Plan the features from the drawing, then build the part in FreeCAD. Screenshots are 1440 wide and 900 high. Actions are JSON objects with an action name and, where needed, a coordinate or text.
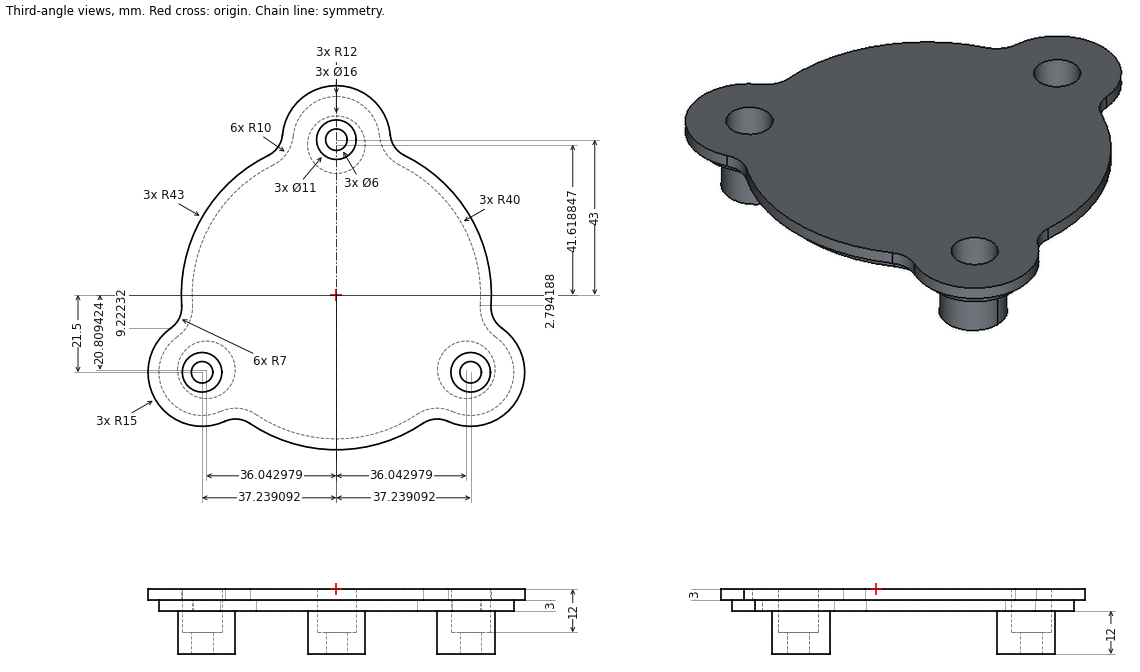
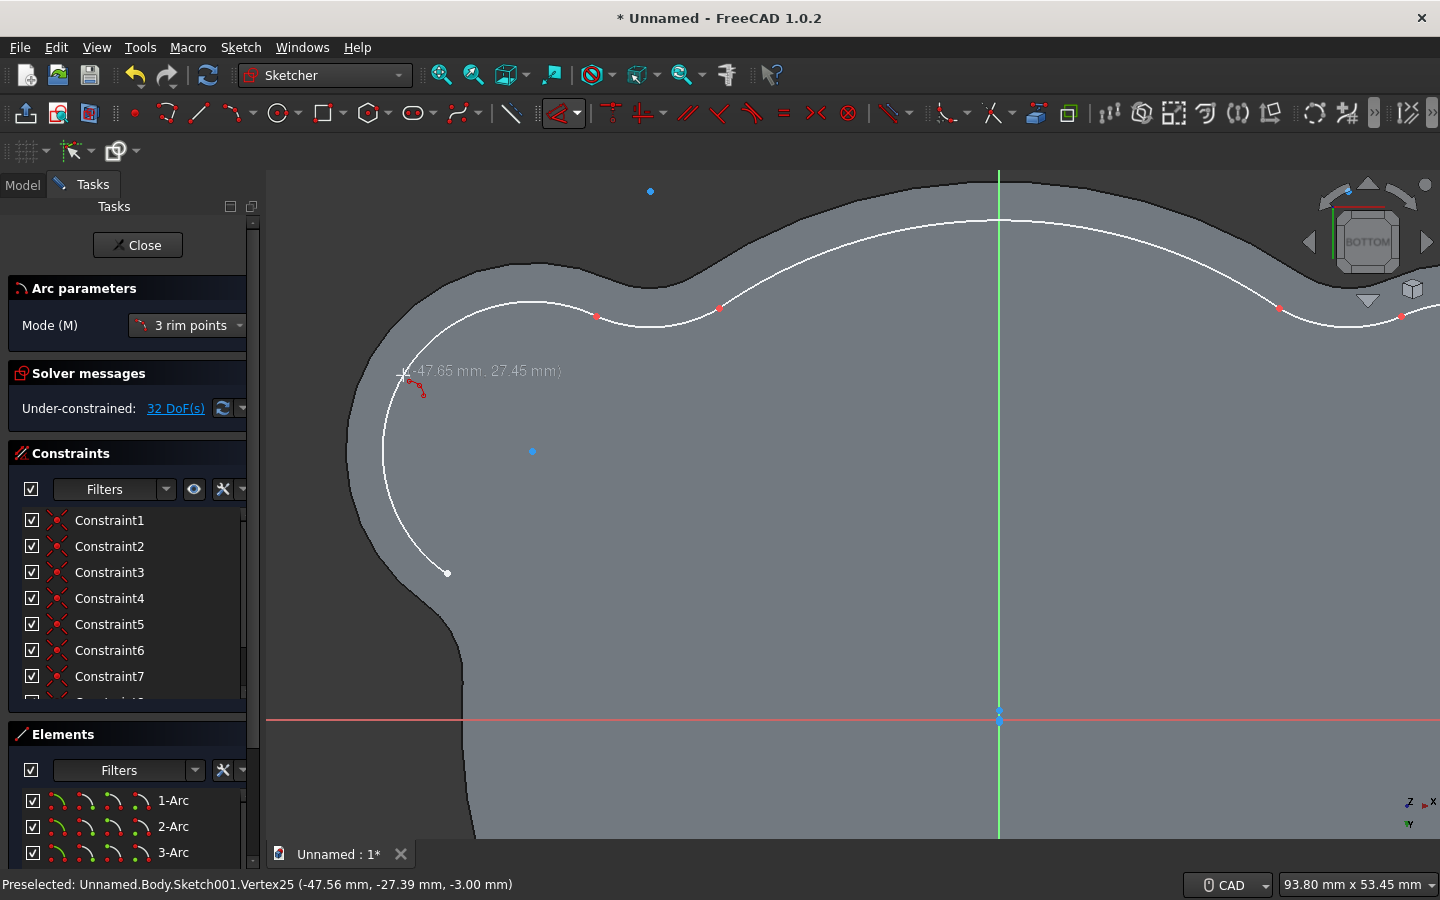
{"action": "left_click", "coordinate": [447, 574]}
{"action": "left_click", "coordinate": [500, 685]}
{"action": "left_click", "coordinate": [488, 622]}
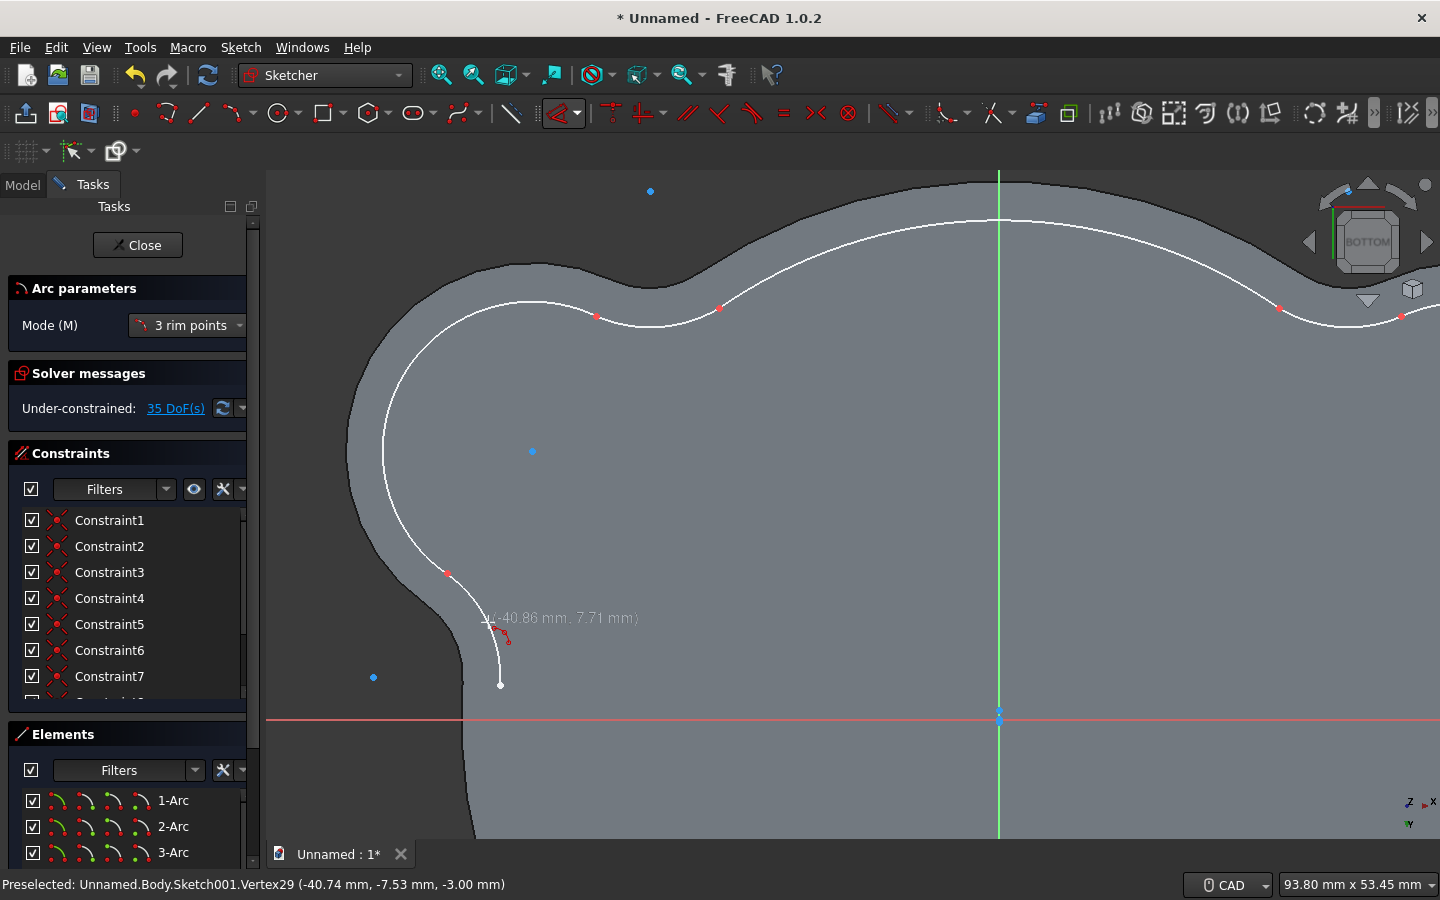
{"action": "left_click", "coordinate": [500, 686]}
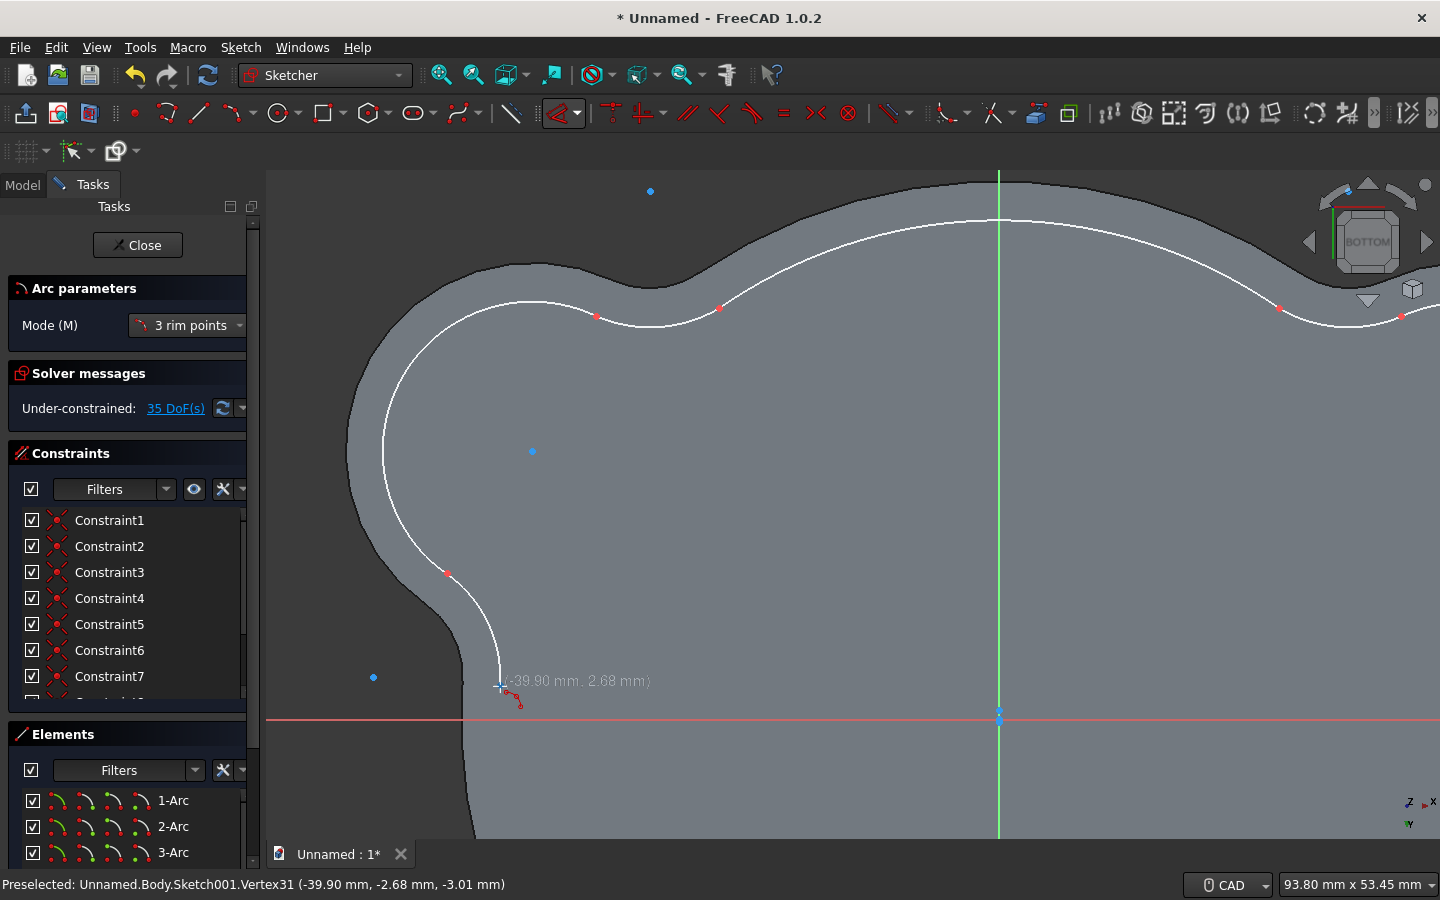
{"action": "scroll", "coordinate": [659, 325], "scroll_direction": "down", "scroll_amount": 5}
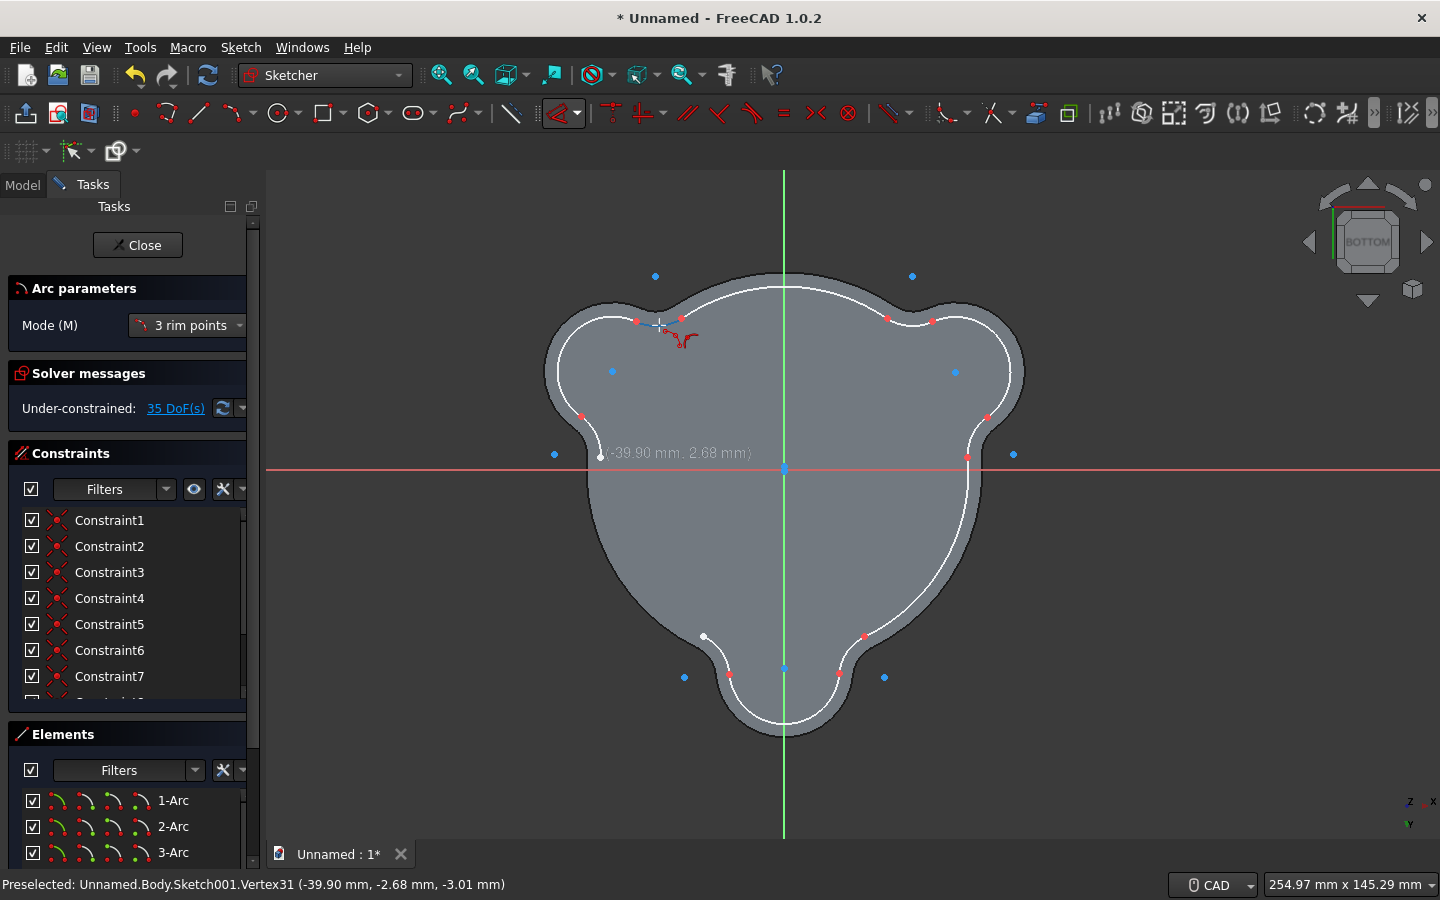
{"action": "left_click", "coordinate": [703, 636]}
{"action": "left_click", "coordinate": [625, 562]}
{"action": "key", "text": "Escape"}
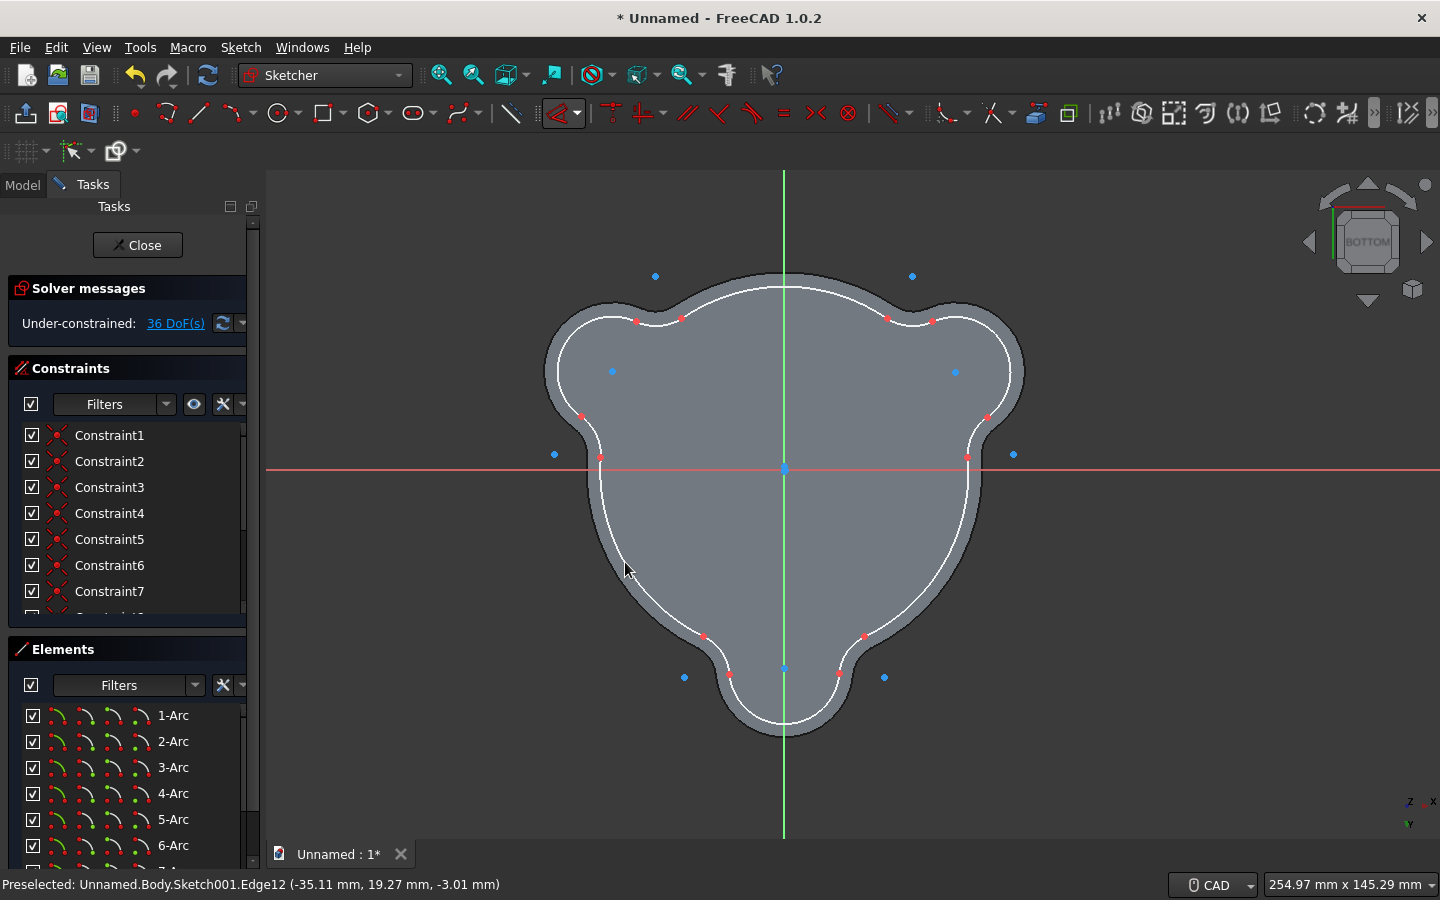
{"action": "left_click", "coordinate": [726, 660]}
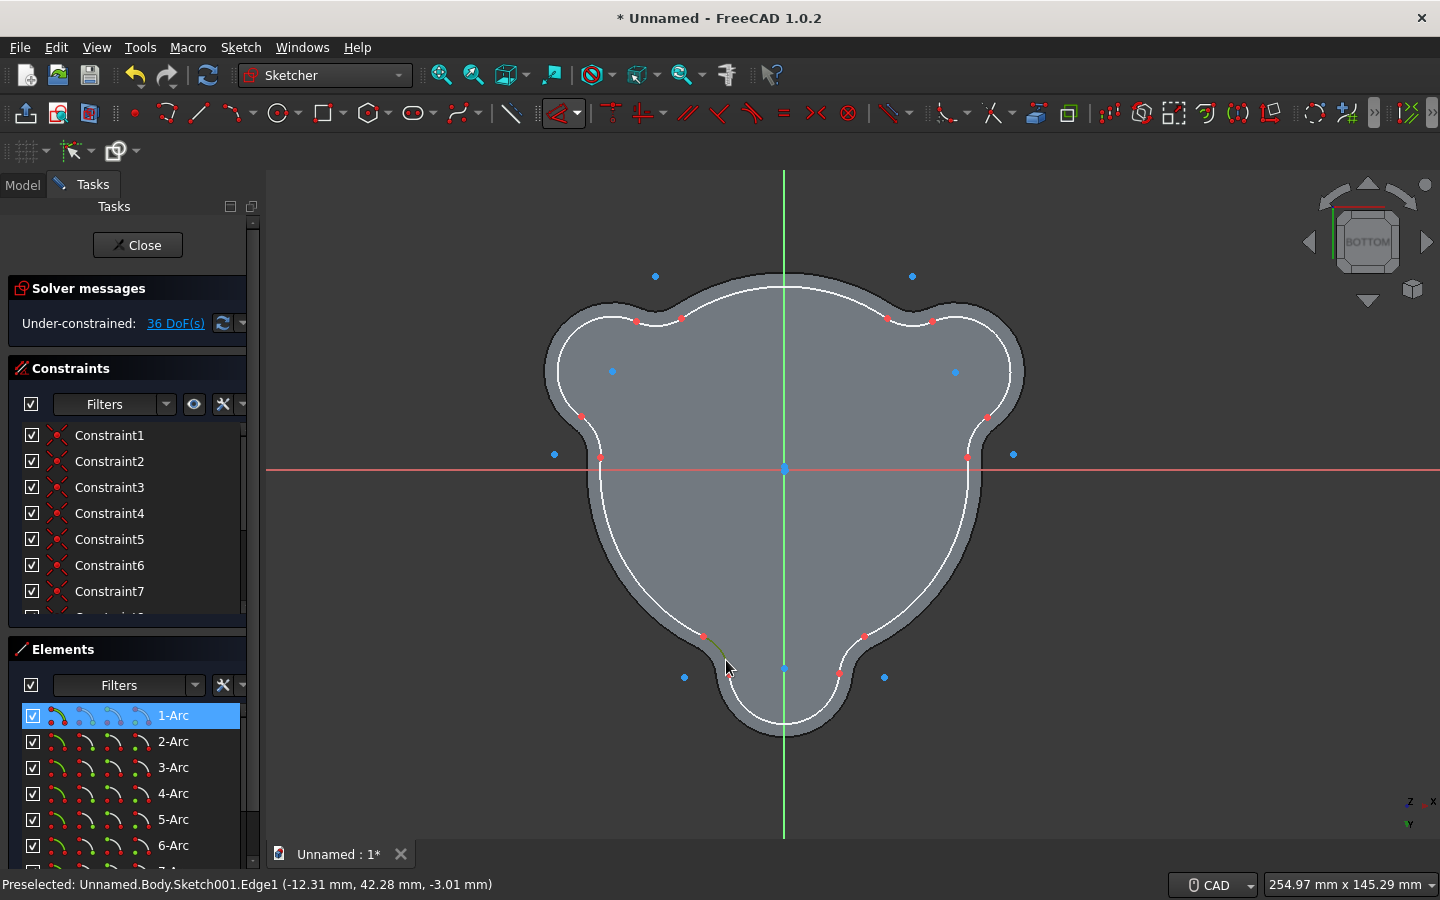
{"action": "left_click", "coordinate": [754, 715]}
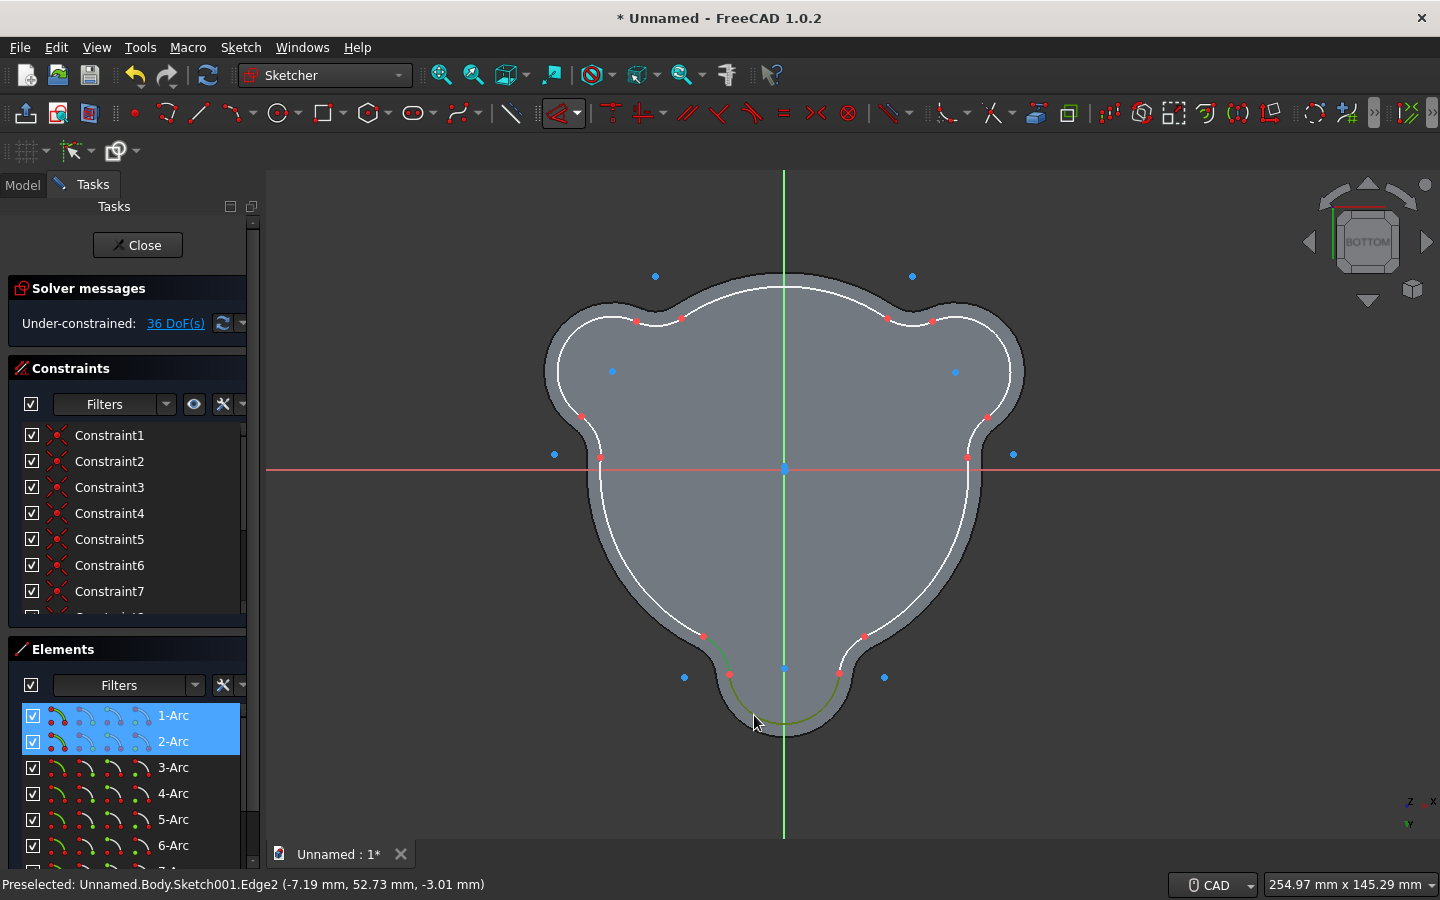
{"action": "left_click", "coordinate": [752, 114]}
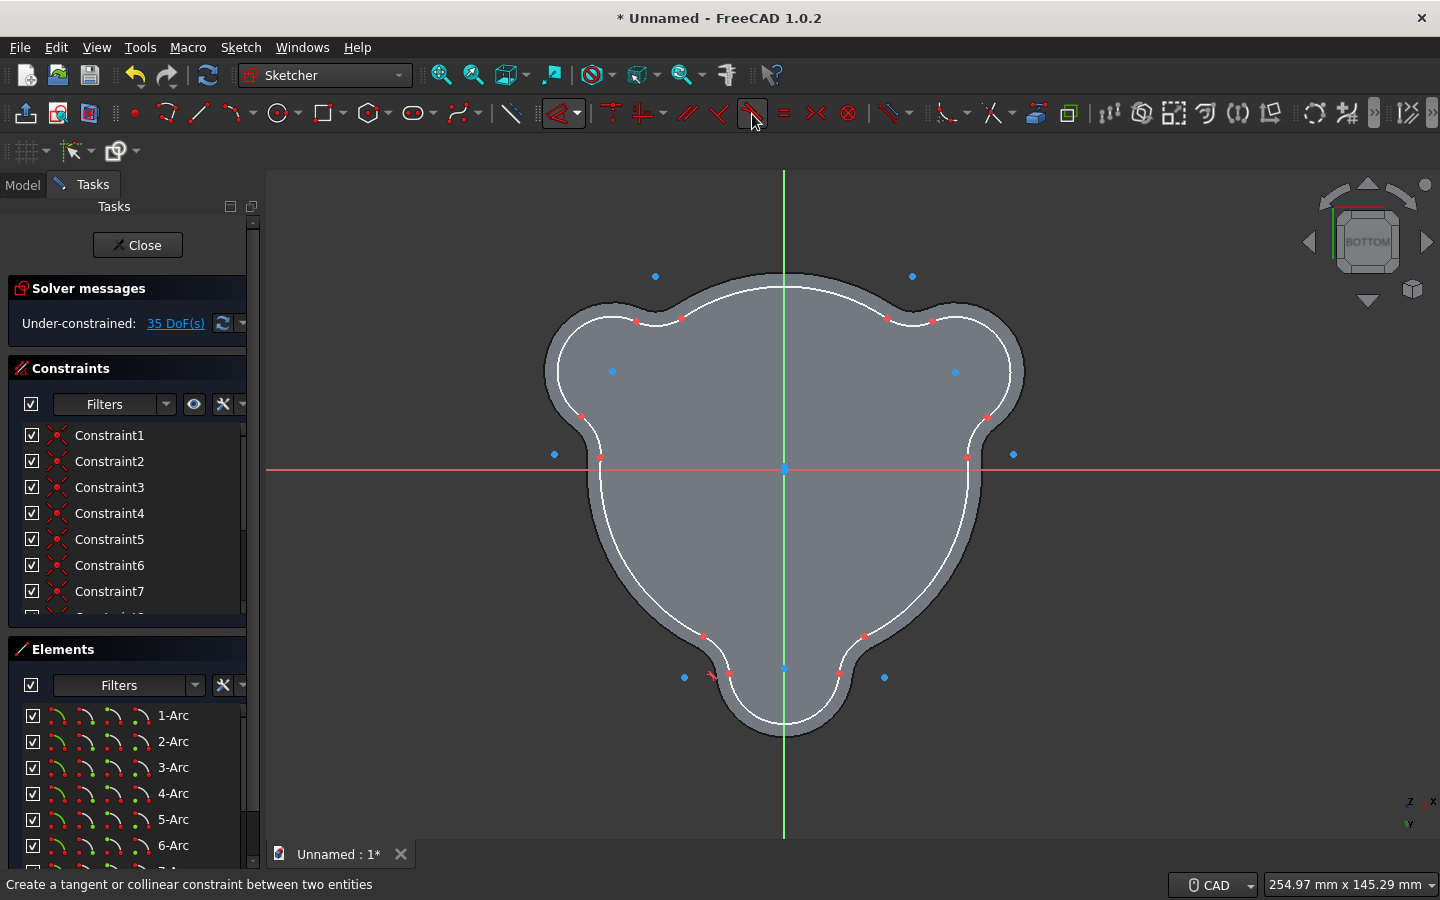
{"action": "left_click", "coordinate": [726, 660]}